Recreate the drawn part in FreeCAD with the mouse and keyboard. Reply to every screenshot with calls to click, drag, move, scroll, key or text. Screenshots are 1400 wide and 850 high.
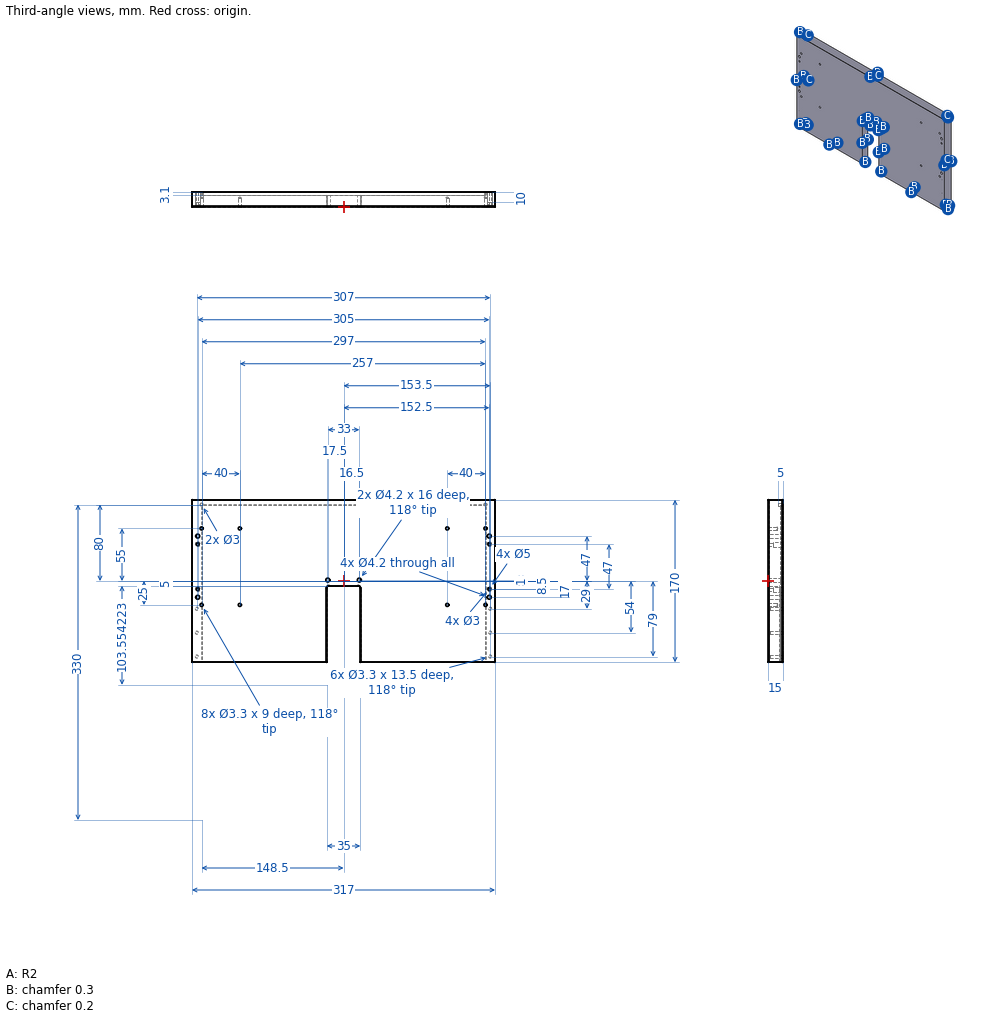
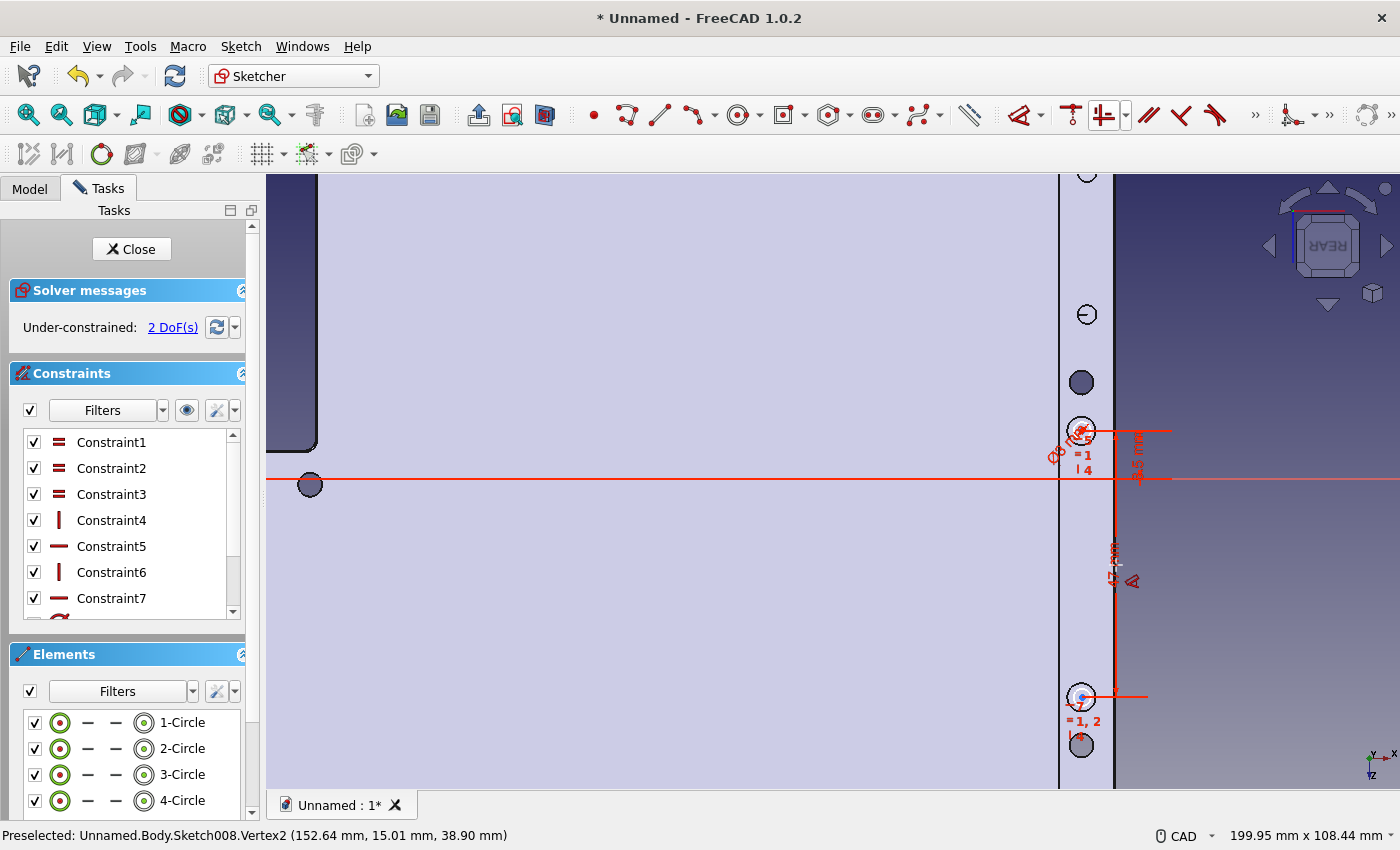
click(1082, 431)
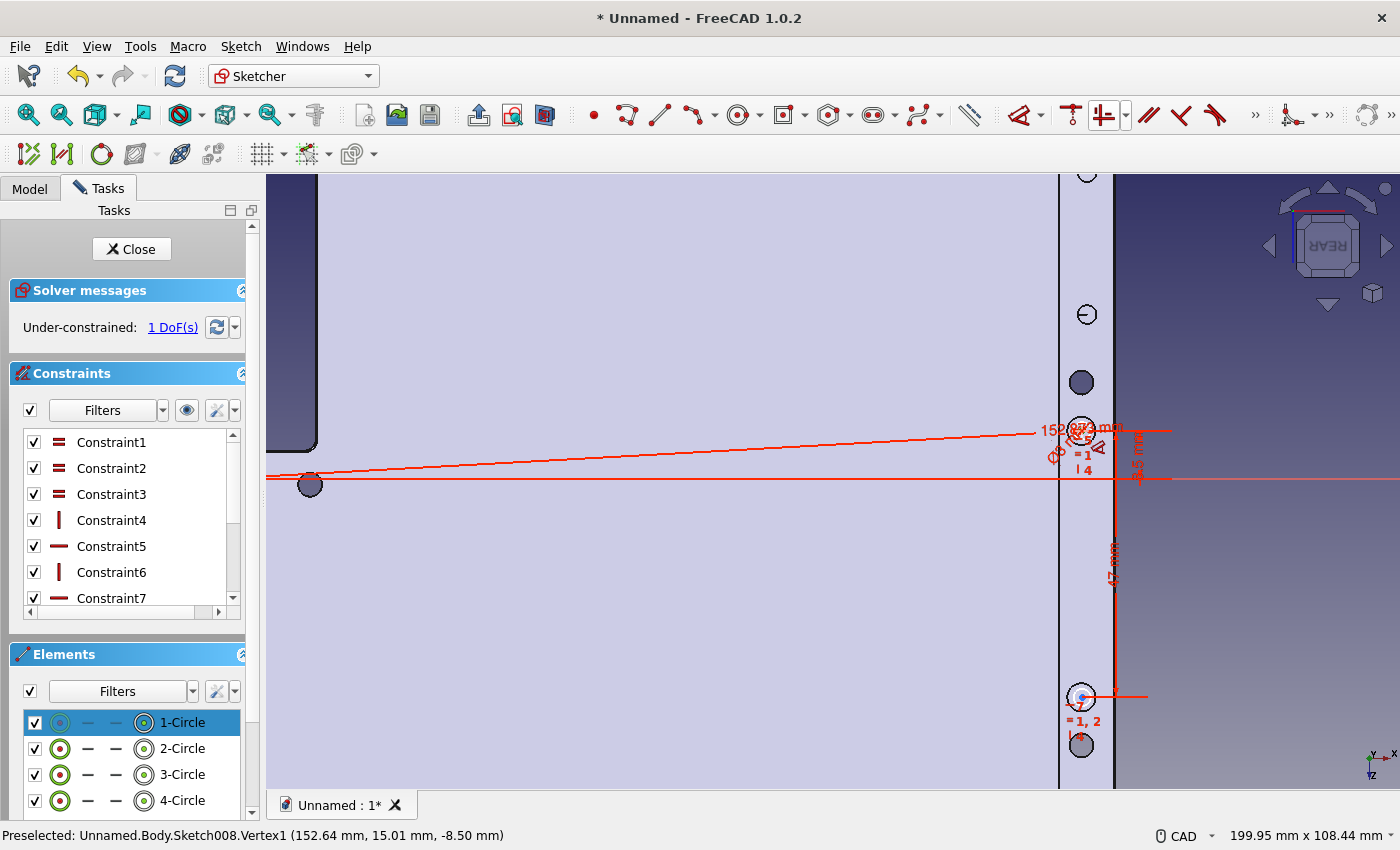
scroll(1083, 433, down, 5)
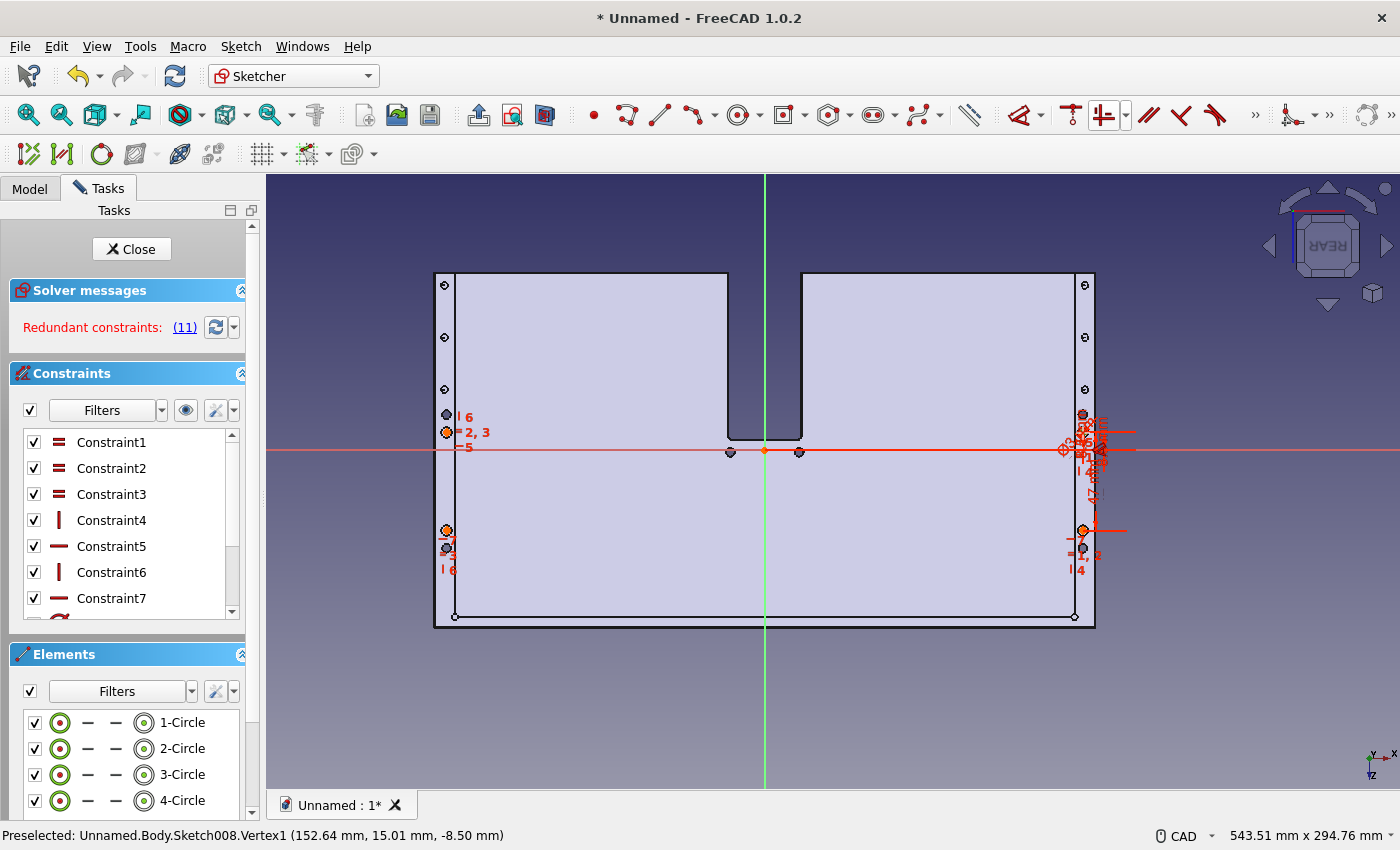
click(447, 432)
click(619, 398)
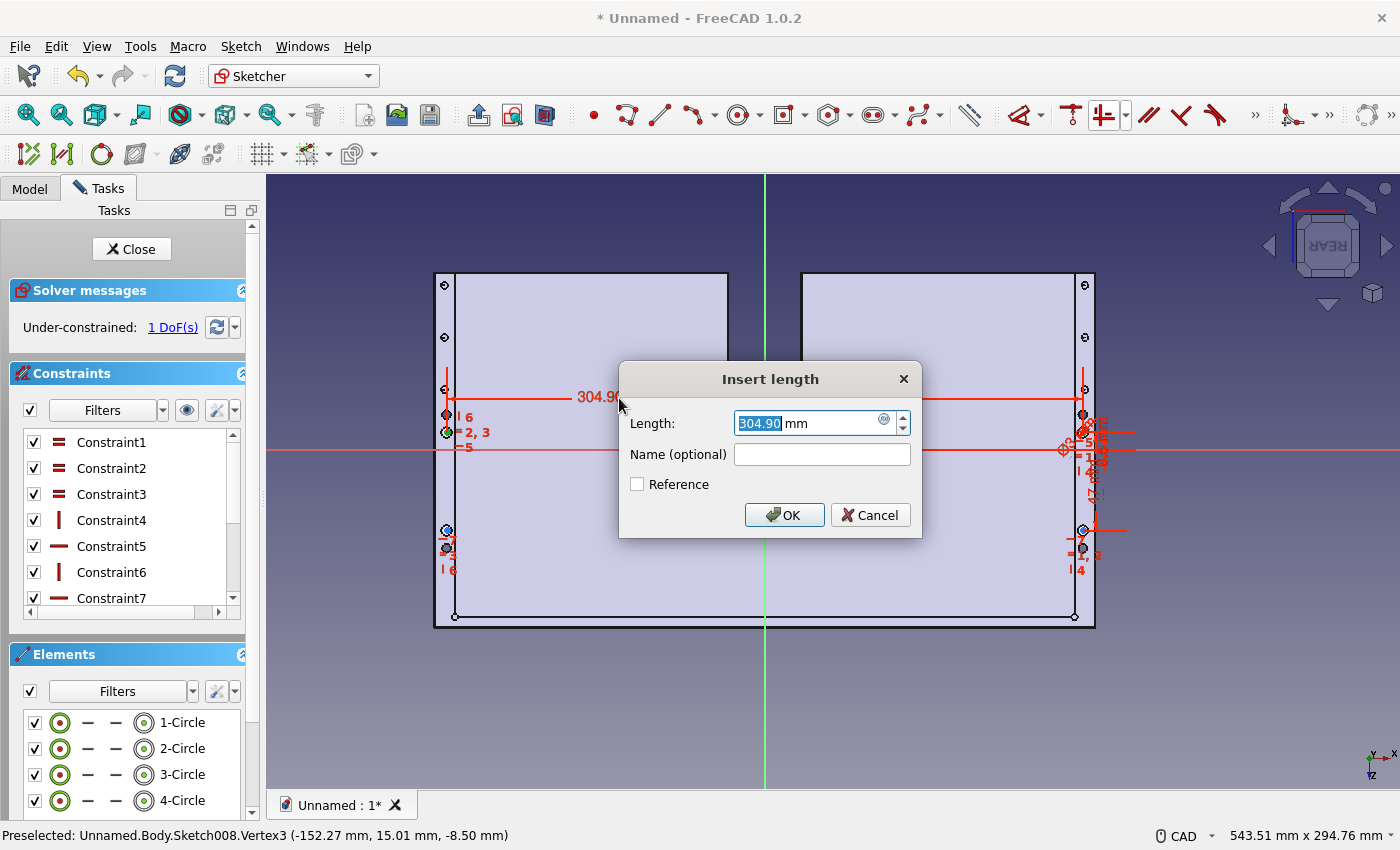
text(305)
key(Return)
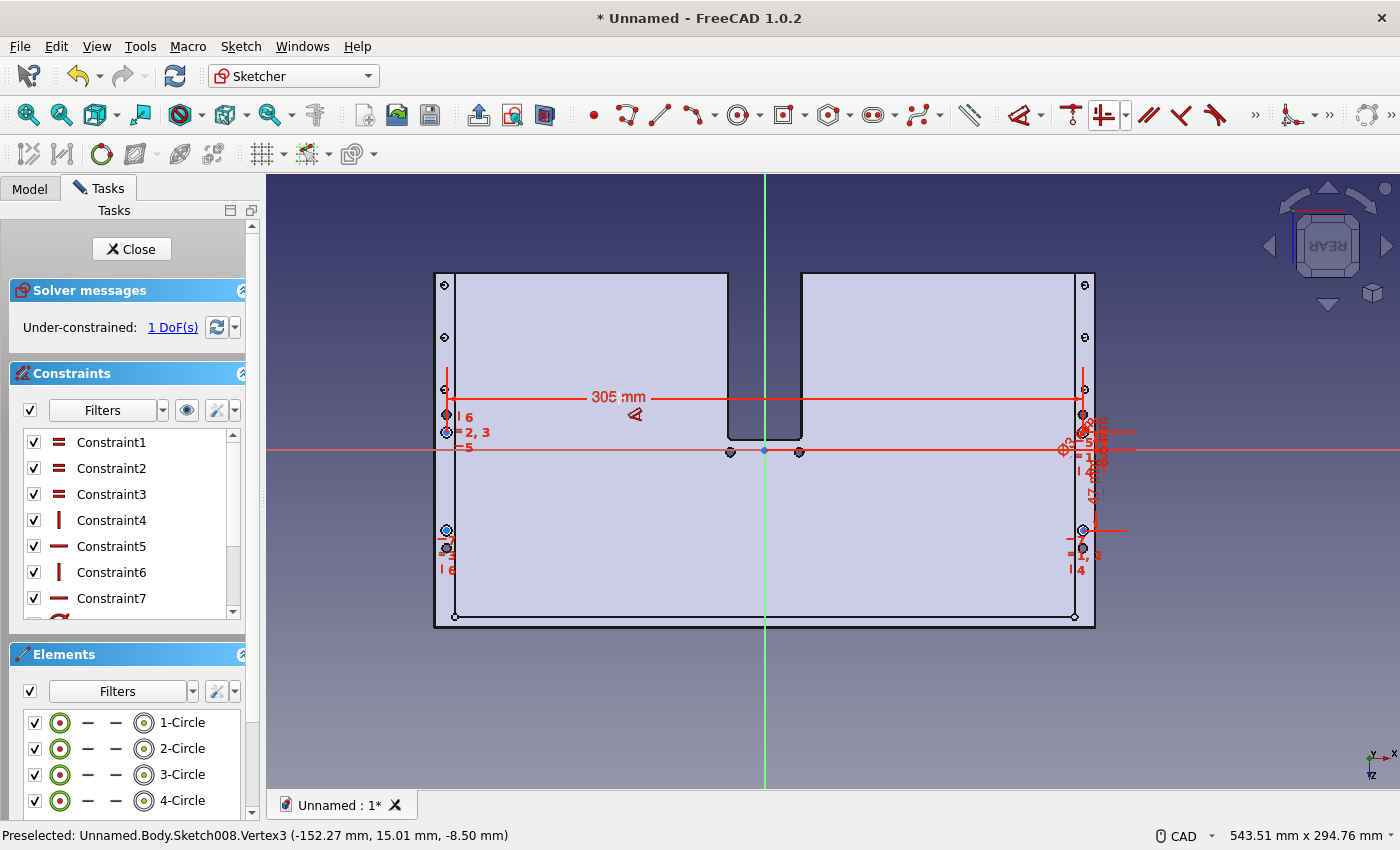
click(1083, 432)
click(924, 398)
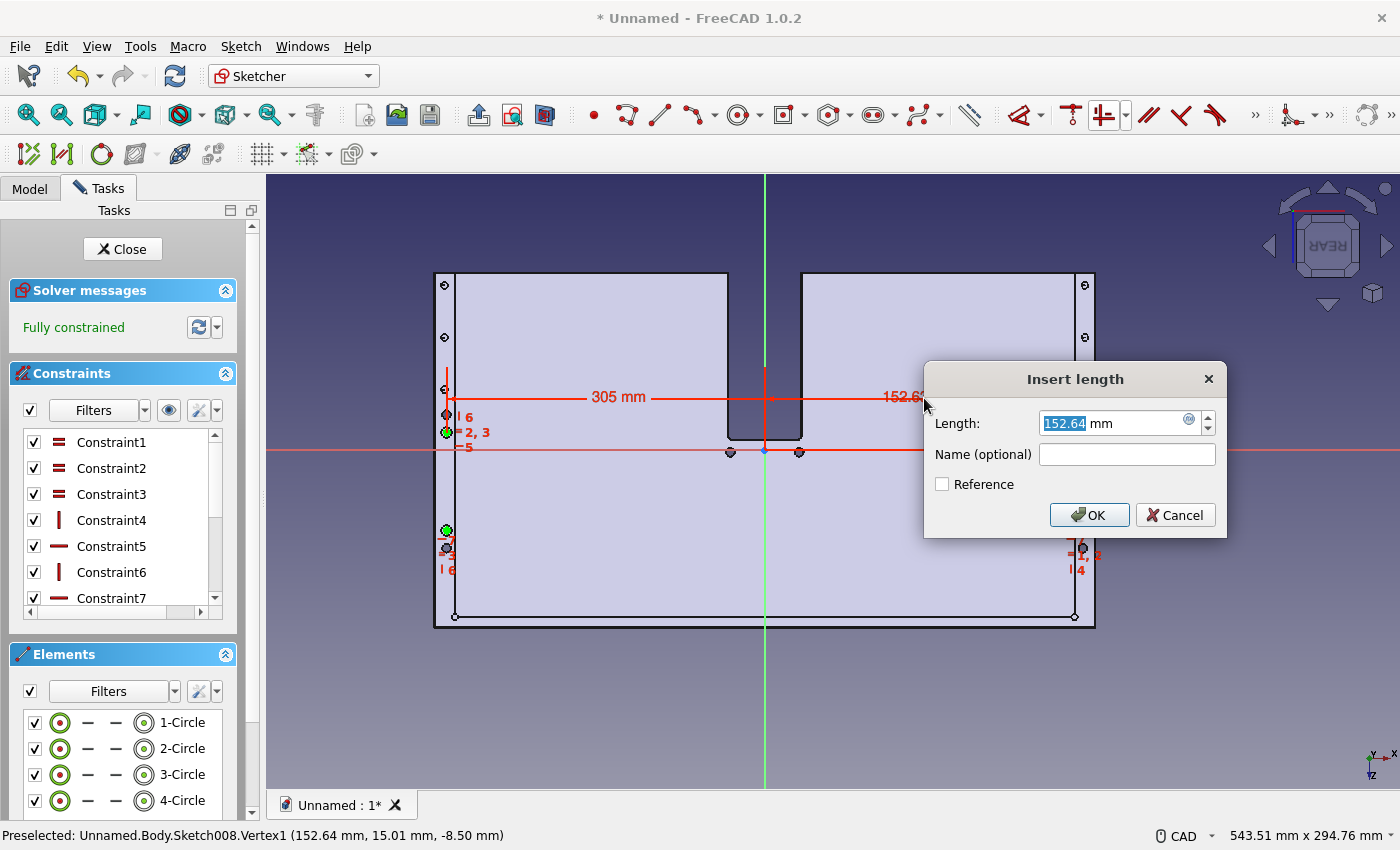
text(152.5)
key(Return)
key(Escape)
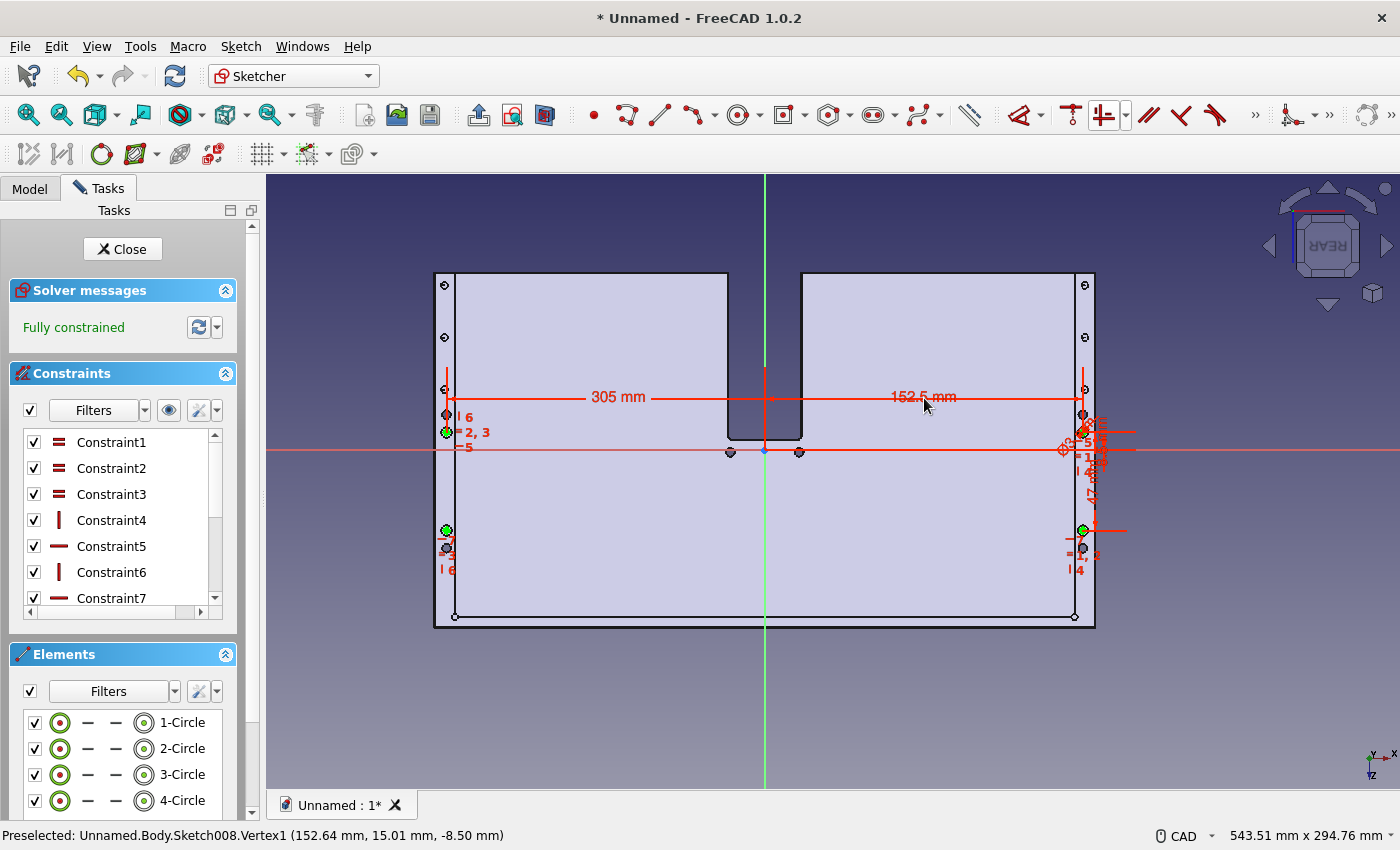
click(123, 249)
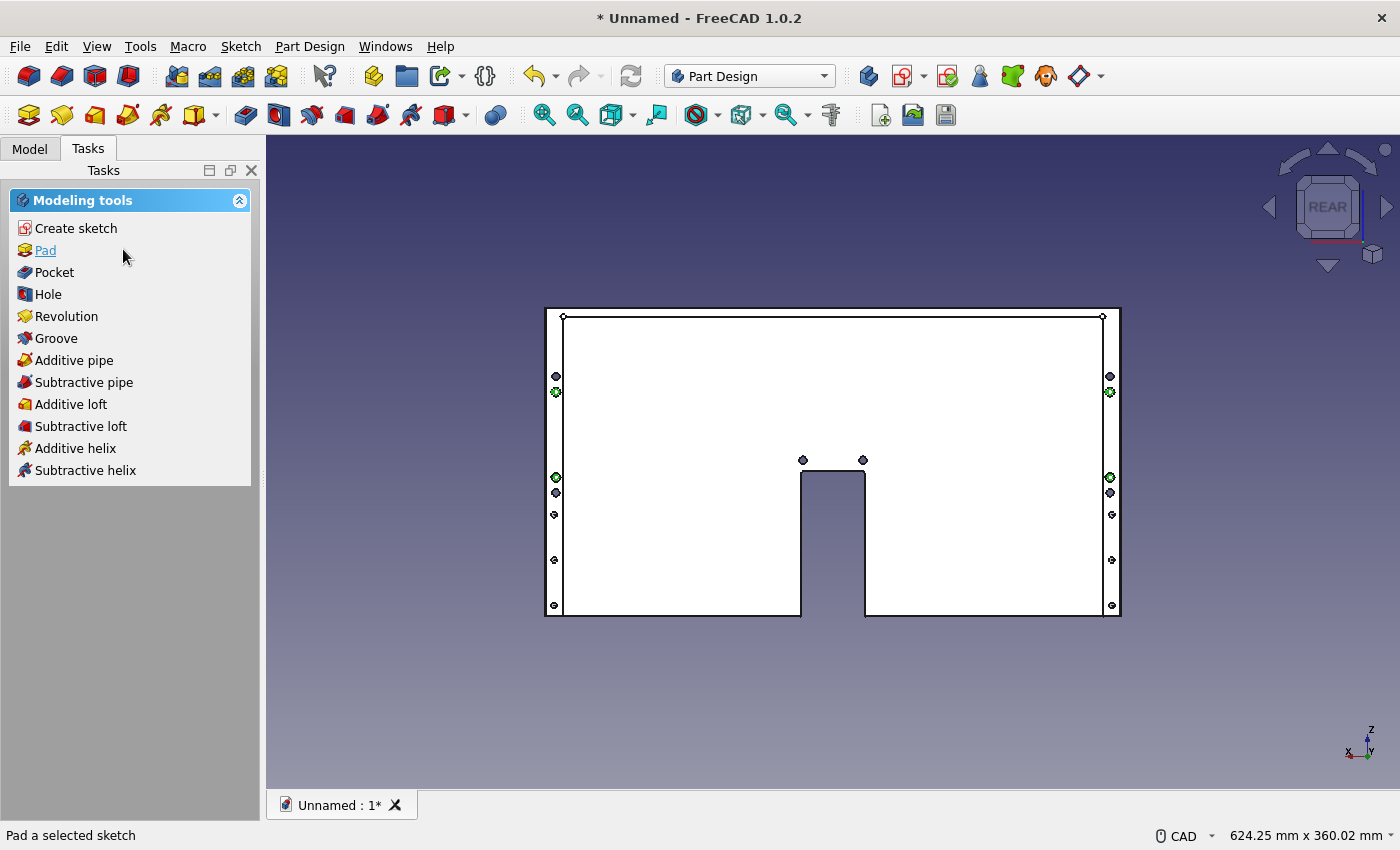
click(246, 116)